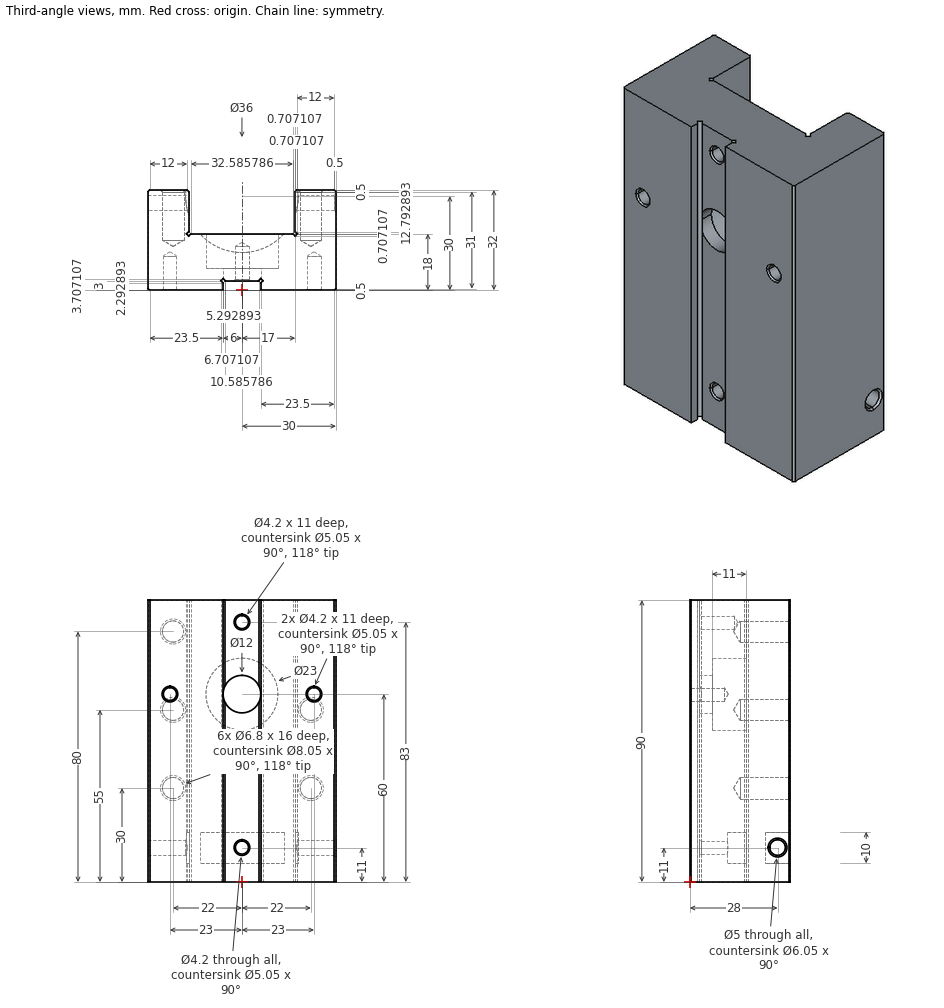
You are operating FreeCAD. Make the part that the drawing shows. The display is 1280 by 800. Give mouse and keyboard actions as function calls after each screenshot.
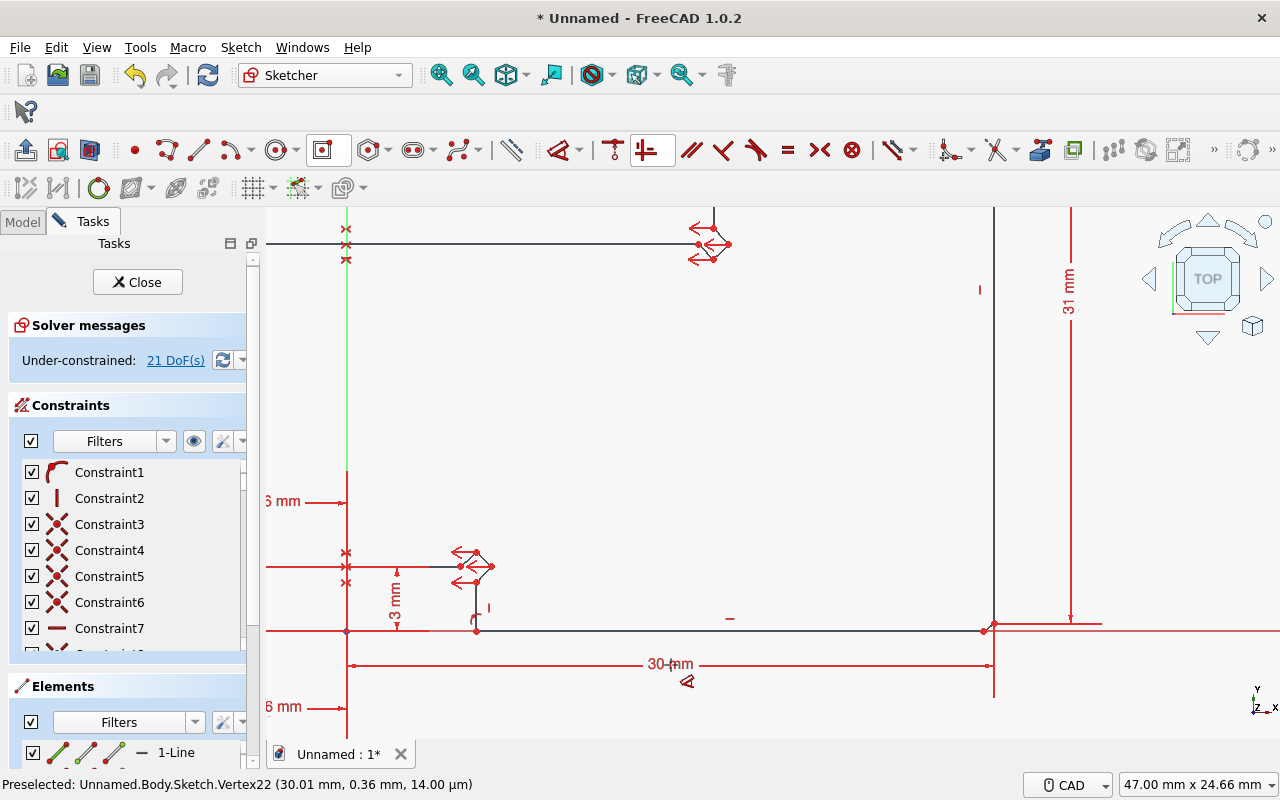
scroll(996, 625, down, 4)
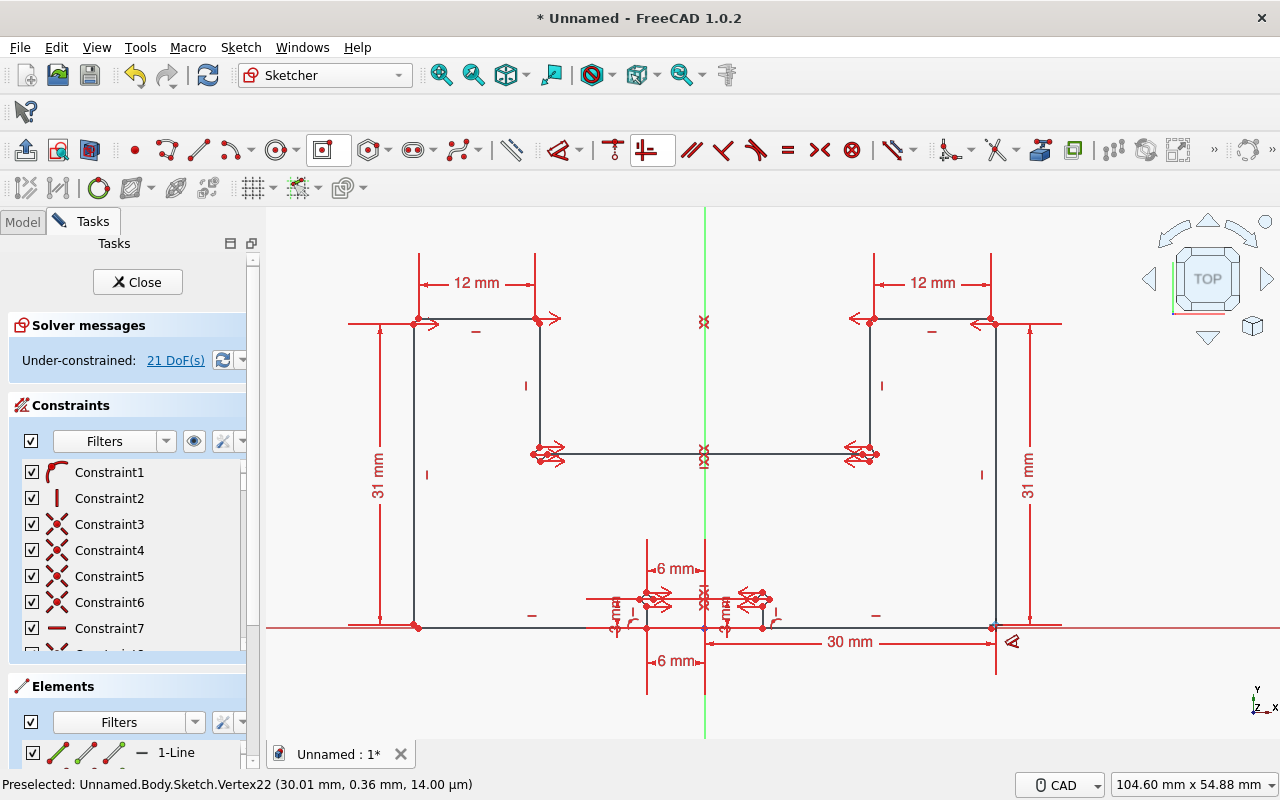
scroll(991, 318, up, 3)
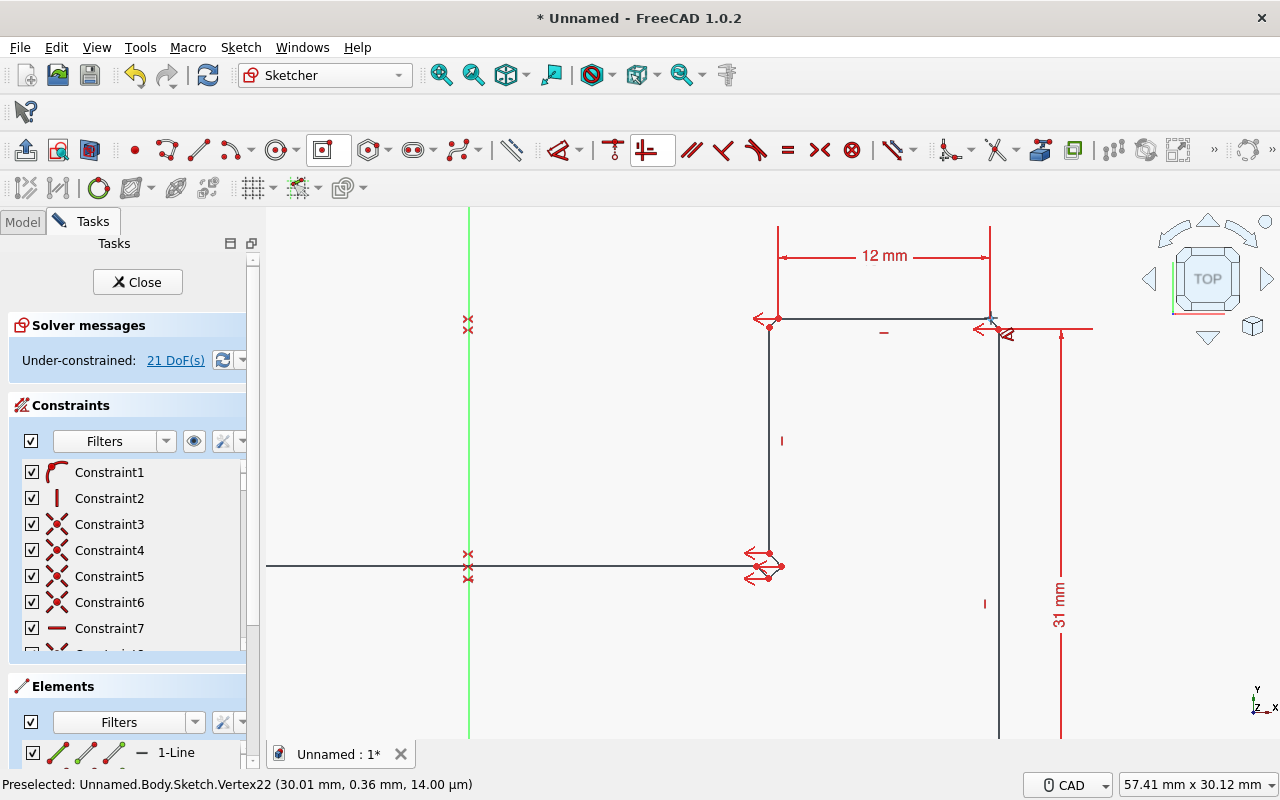
click(990, 319)
click(1024, 515)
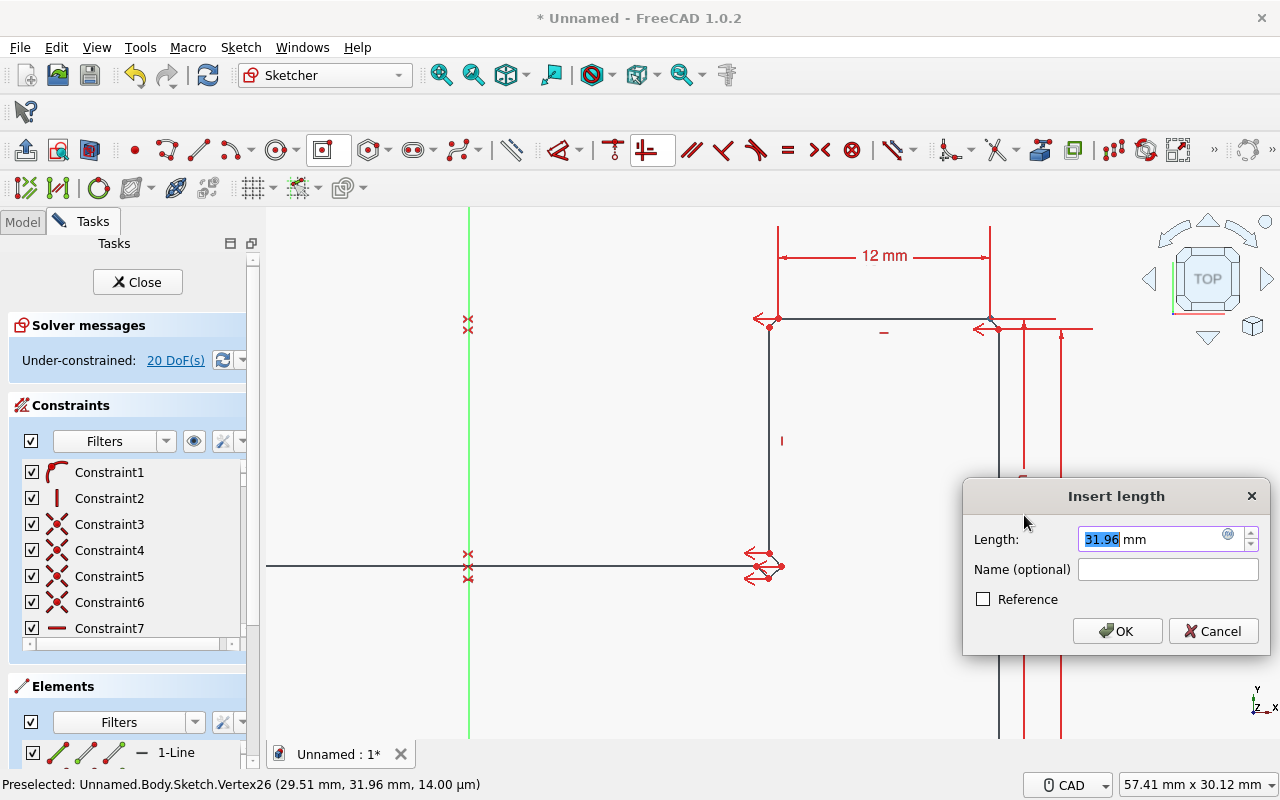
text(32)
key(Return)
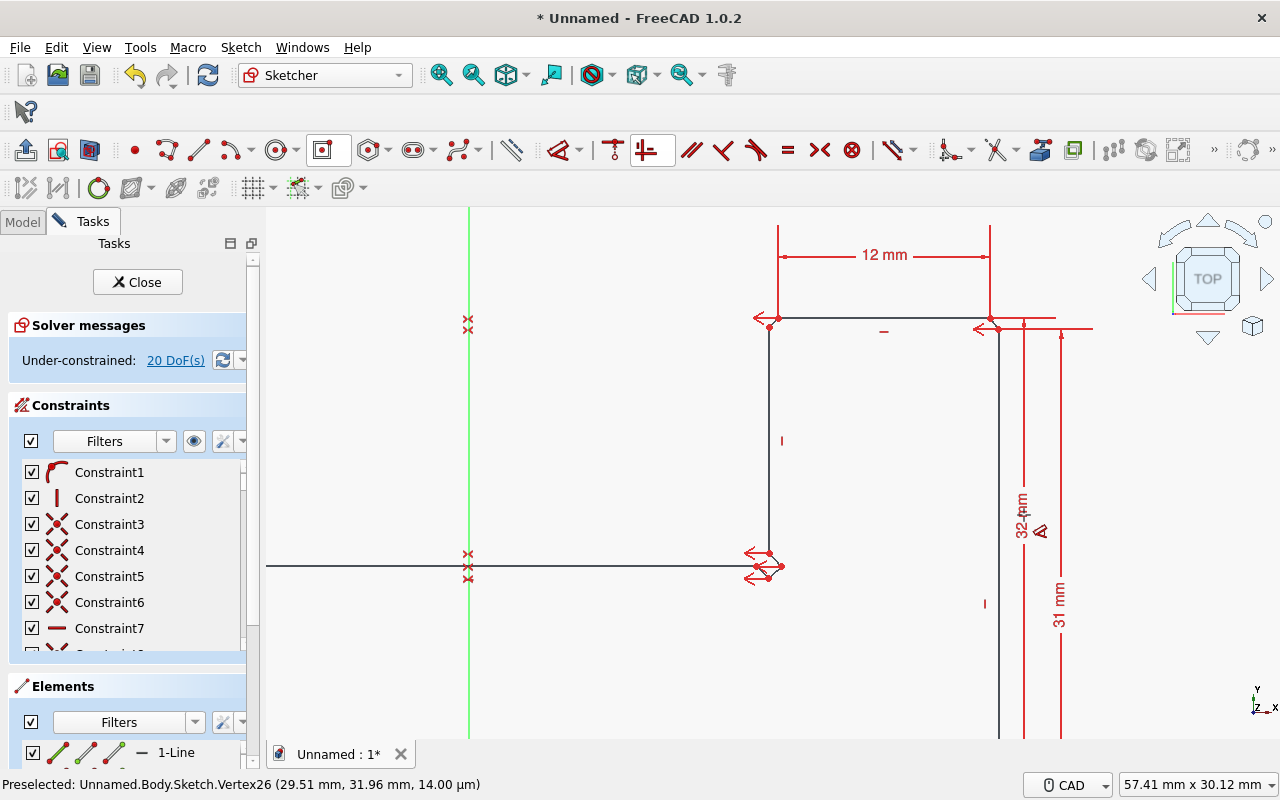
click(769, 327)
click(619, 293)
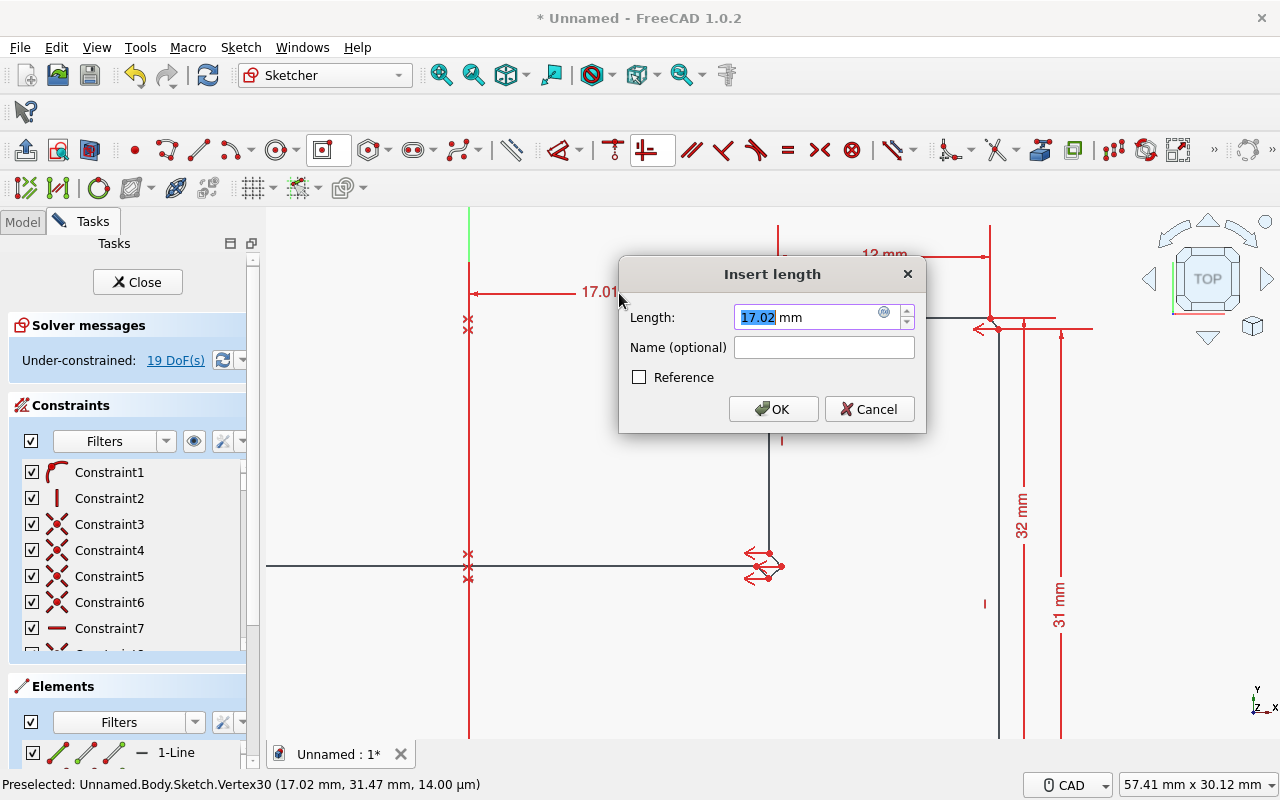
text(17)
key(Return)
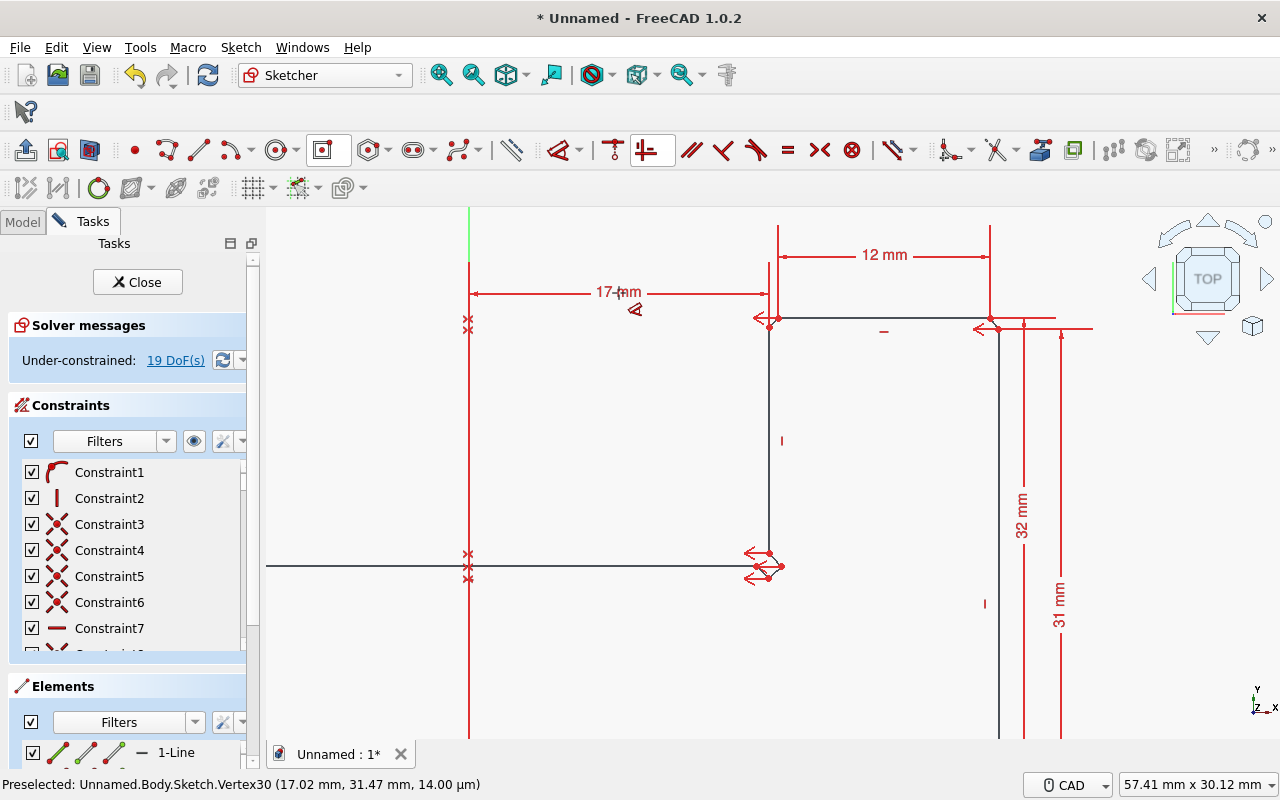
click(781, 567)
click(815, 639)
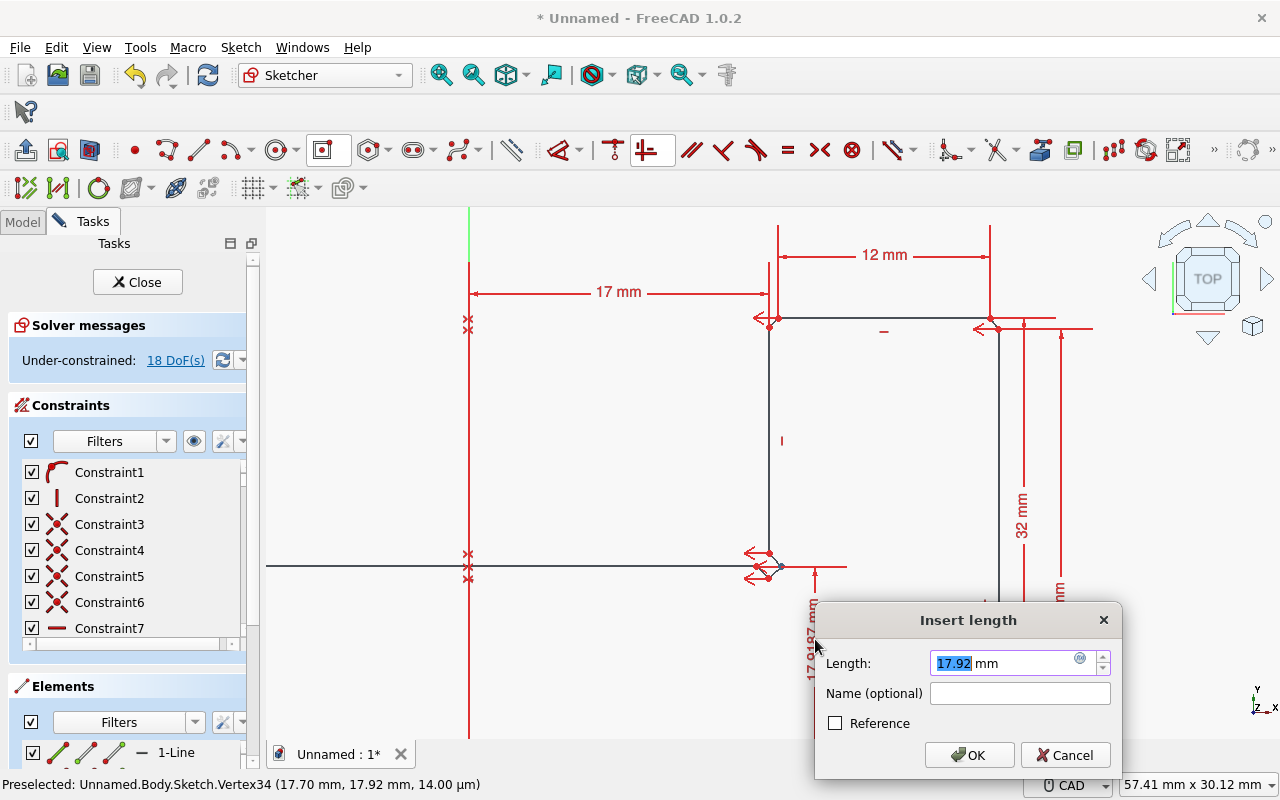
text(18)
key(Return)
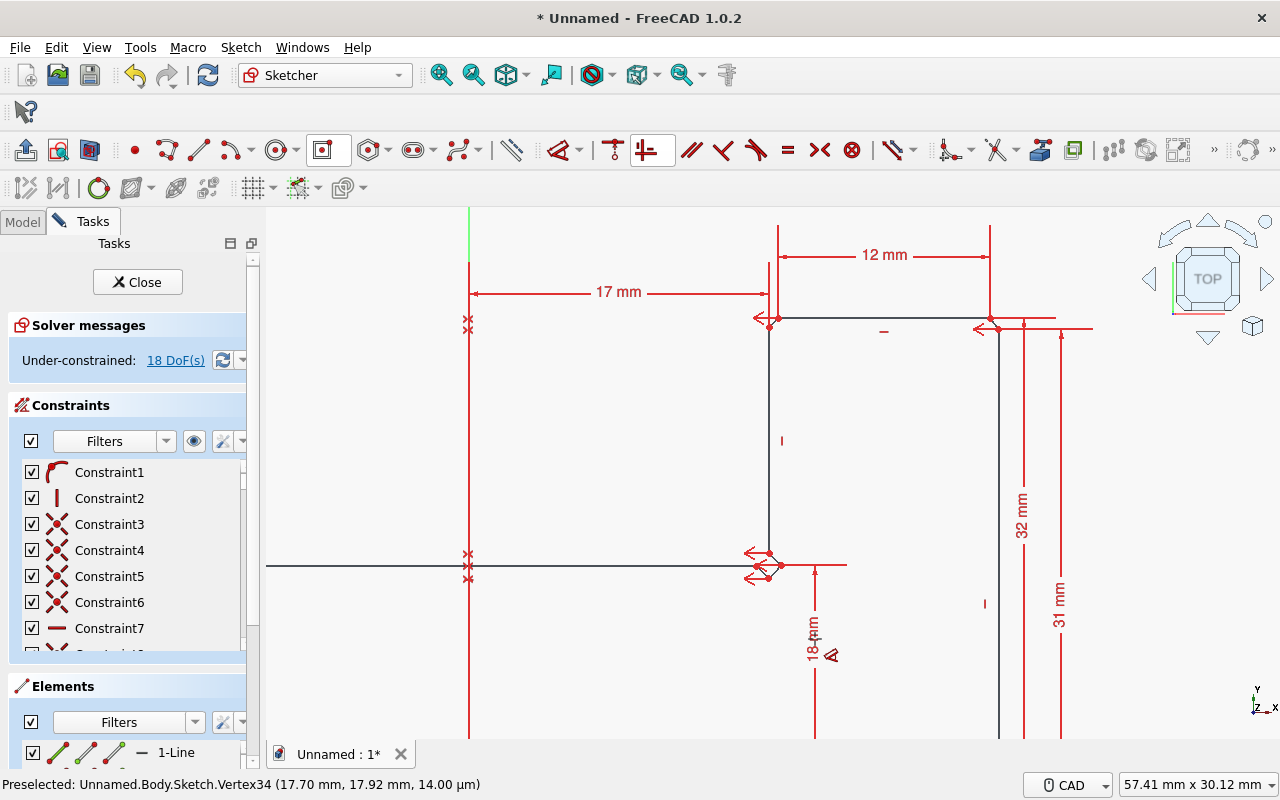
click(769, 579)
click(619, 545)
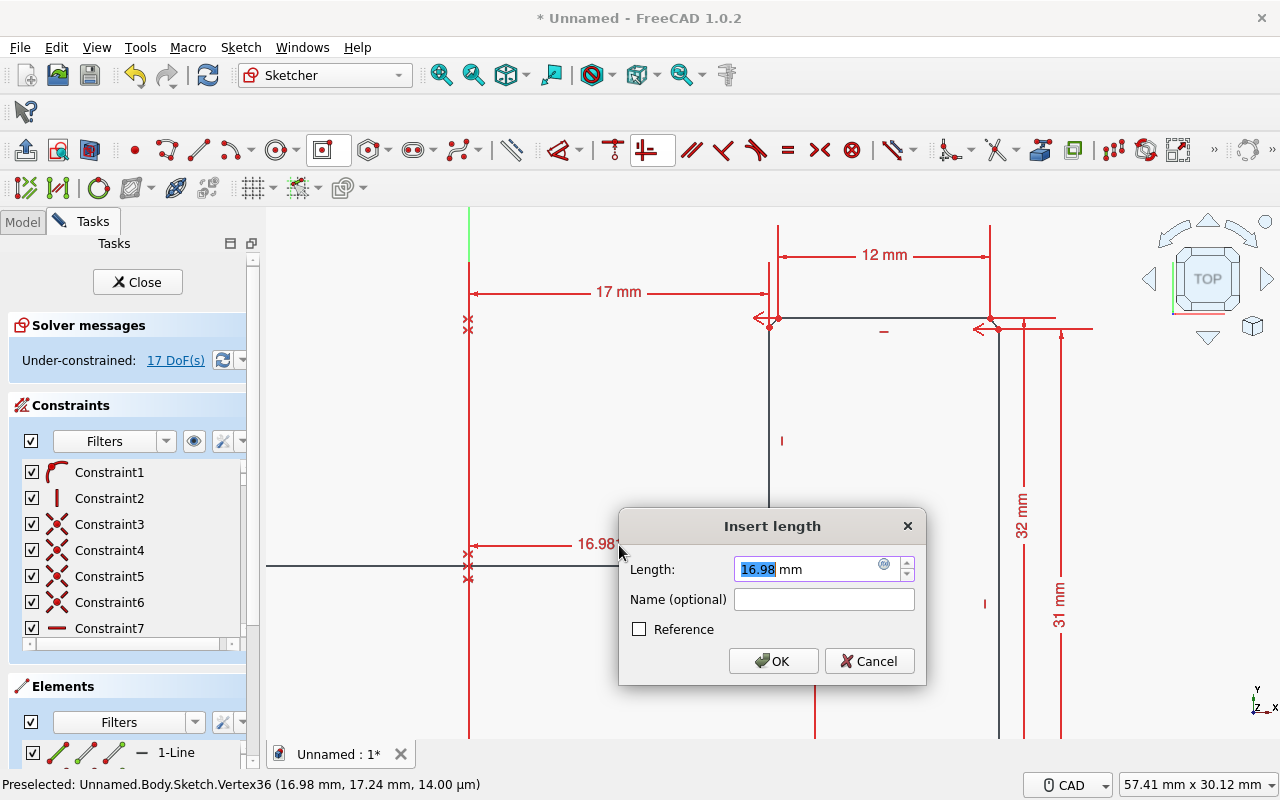
text(17)
key(Return)